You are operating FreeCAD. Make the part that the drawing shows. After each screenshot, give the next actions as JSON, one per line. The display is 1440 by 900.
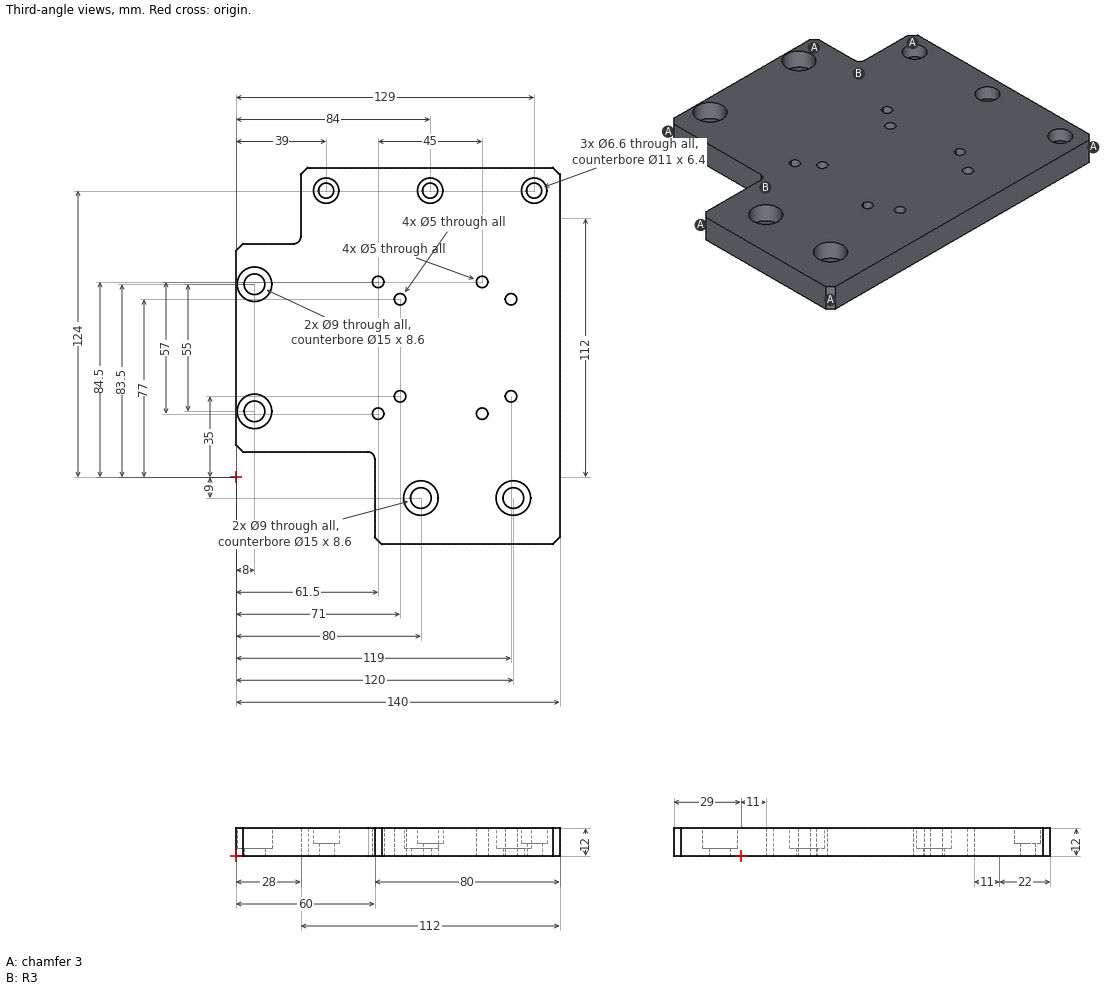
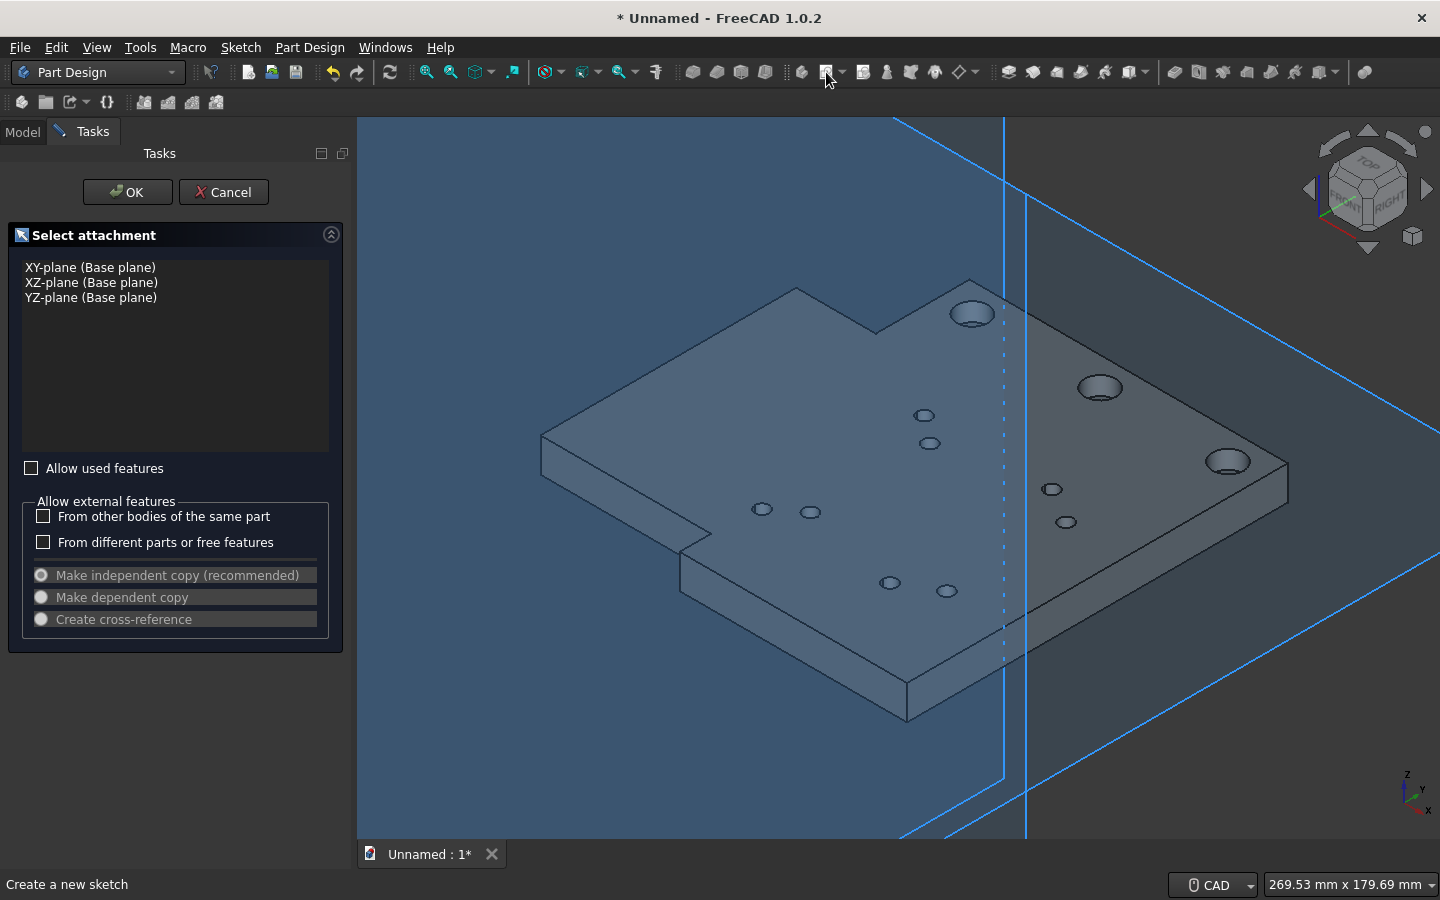
{"action": "left_click", "coordinate": [82, 282]}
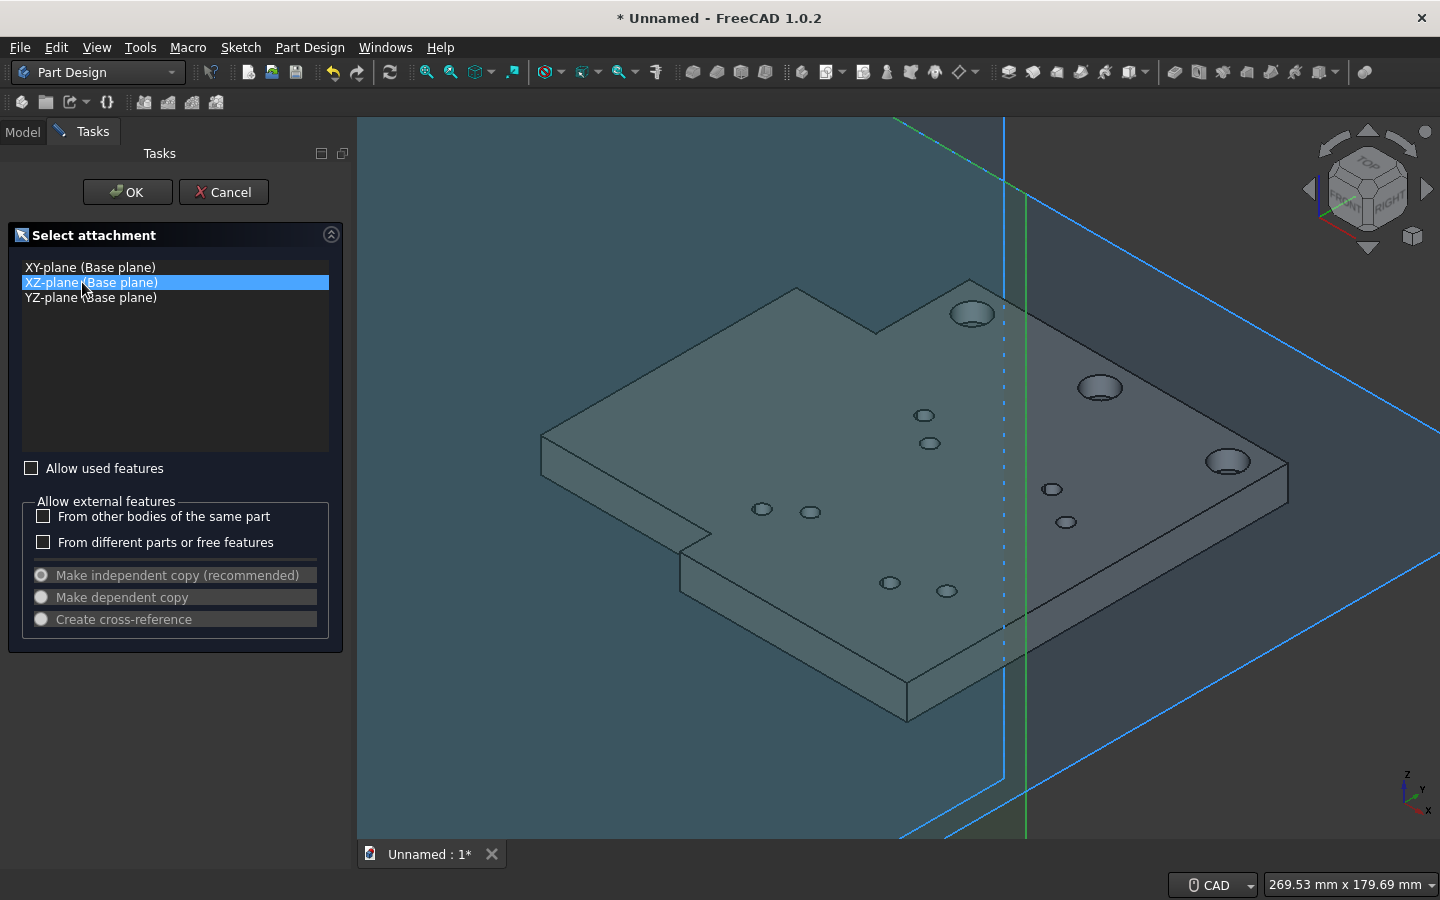
{"action": "left_click", "coordinate": [128, 192]}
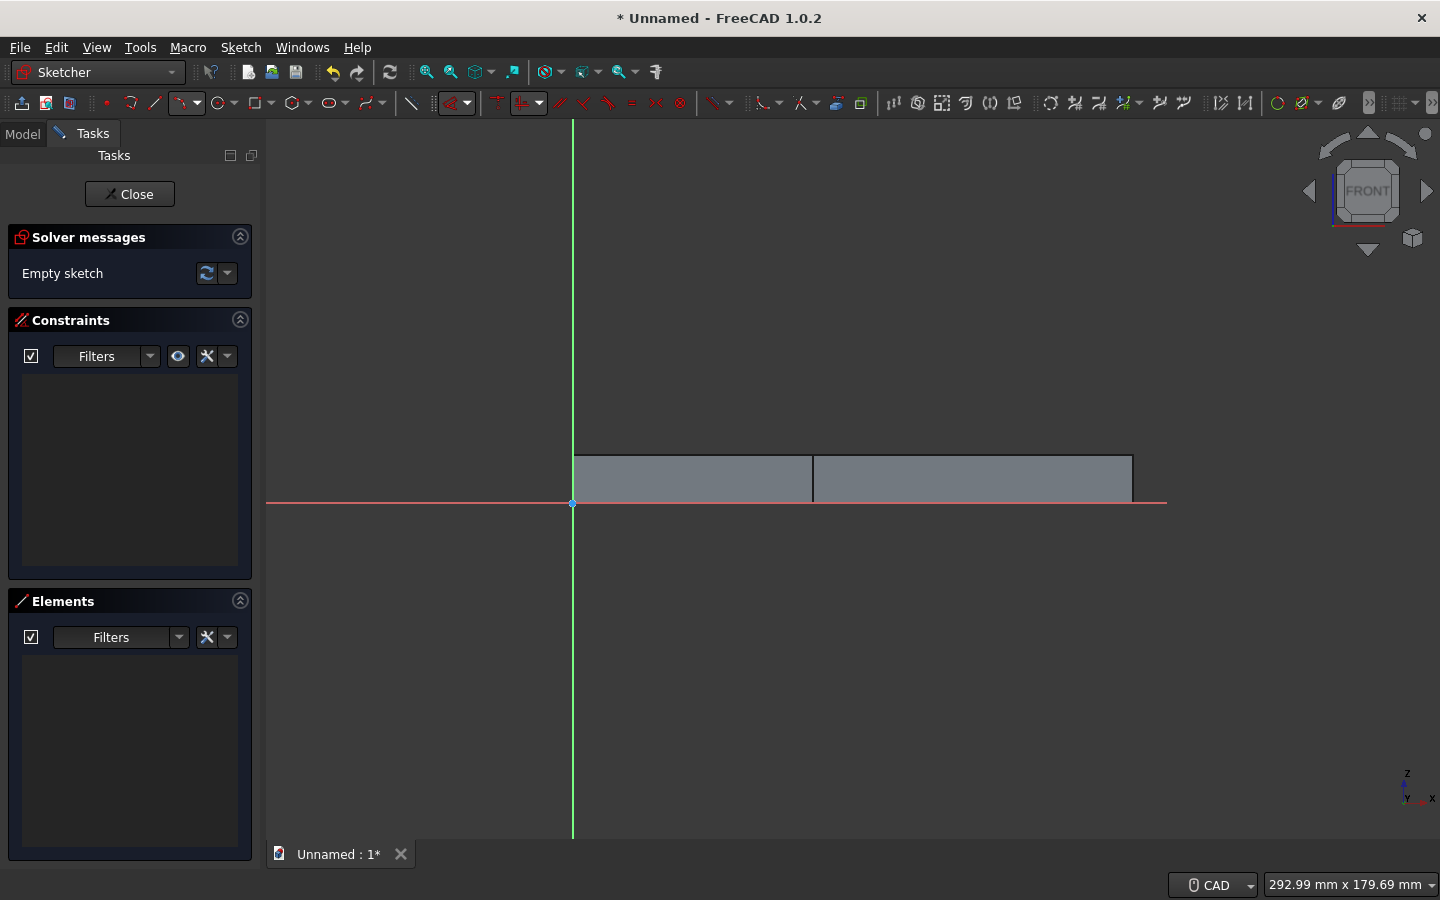
{"action": "left_click", "coordinate": [256, 104]}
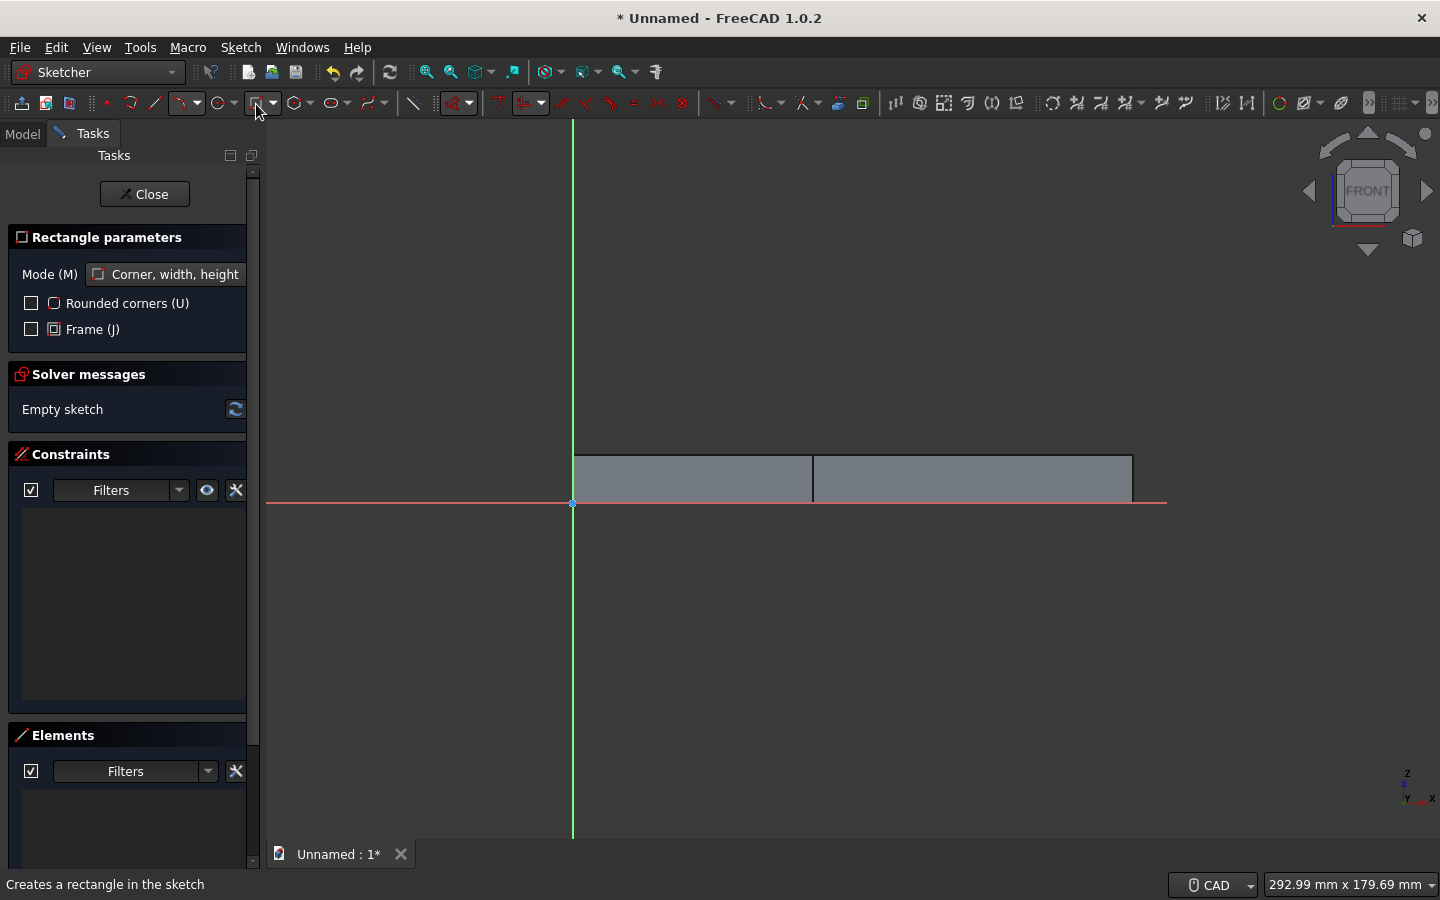
{"action": "left_click", "coordinate": [813, 455]}
{"action": "left_click", "coordinate": [1133, 503]}
{"action": "key", "text": "Escape"}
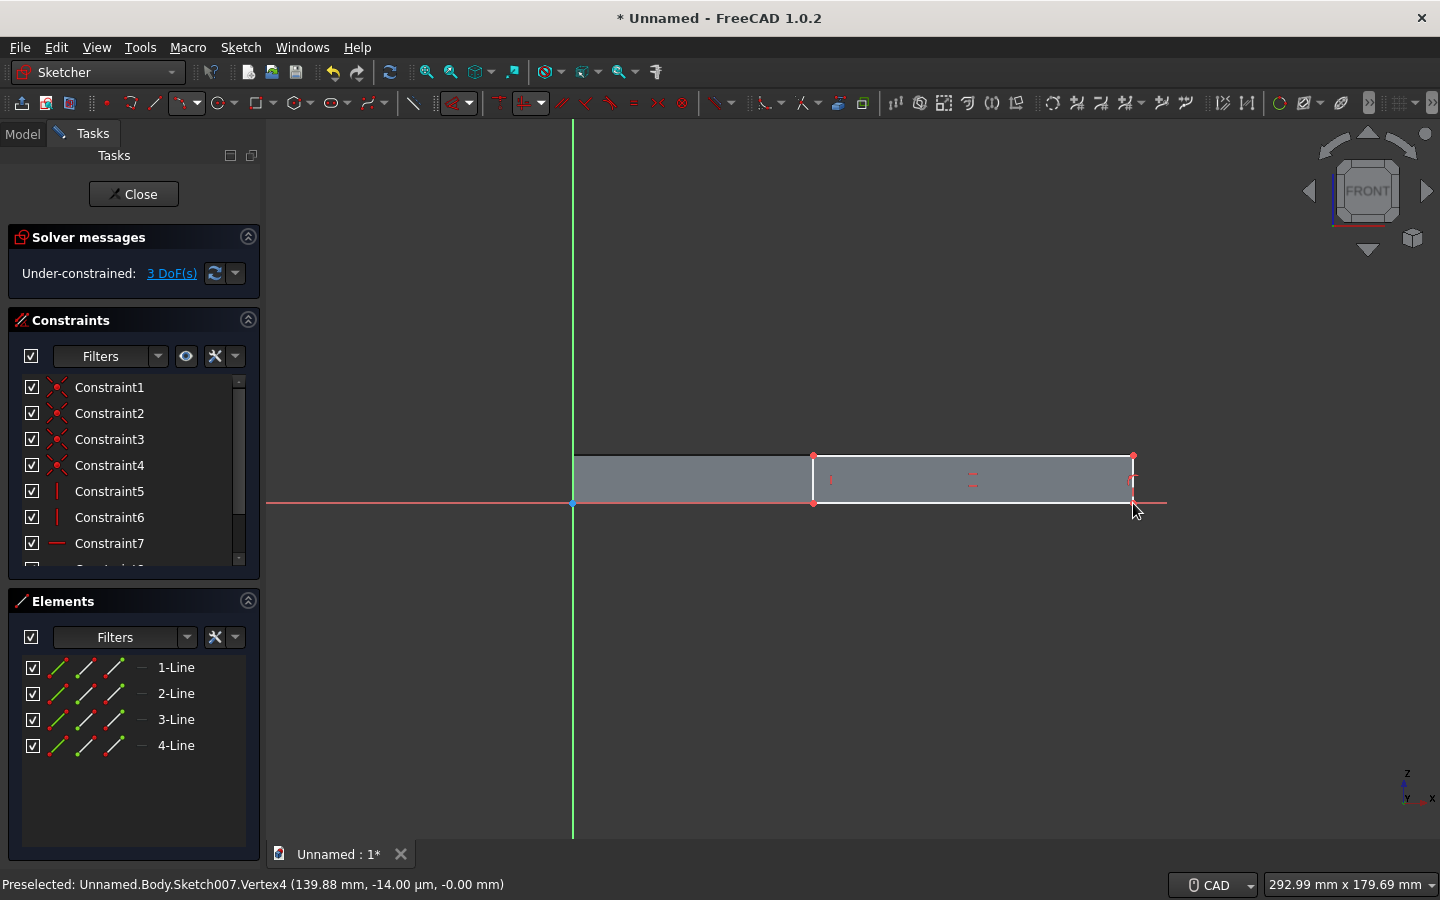
{"action": "left_click", "coordinate": [813, 470]}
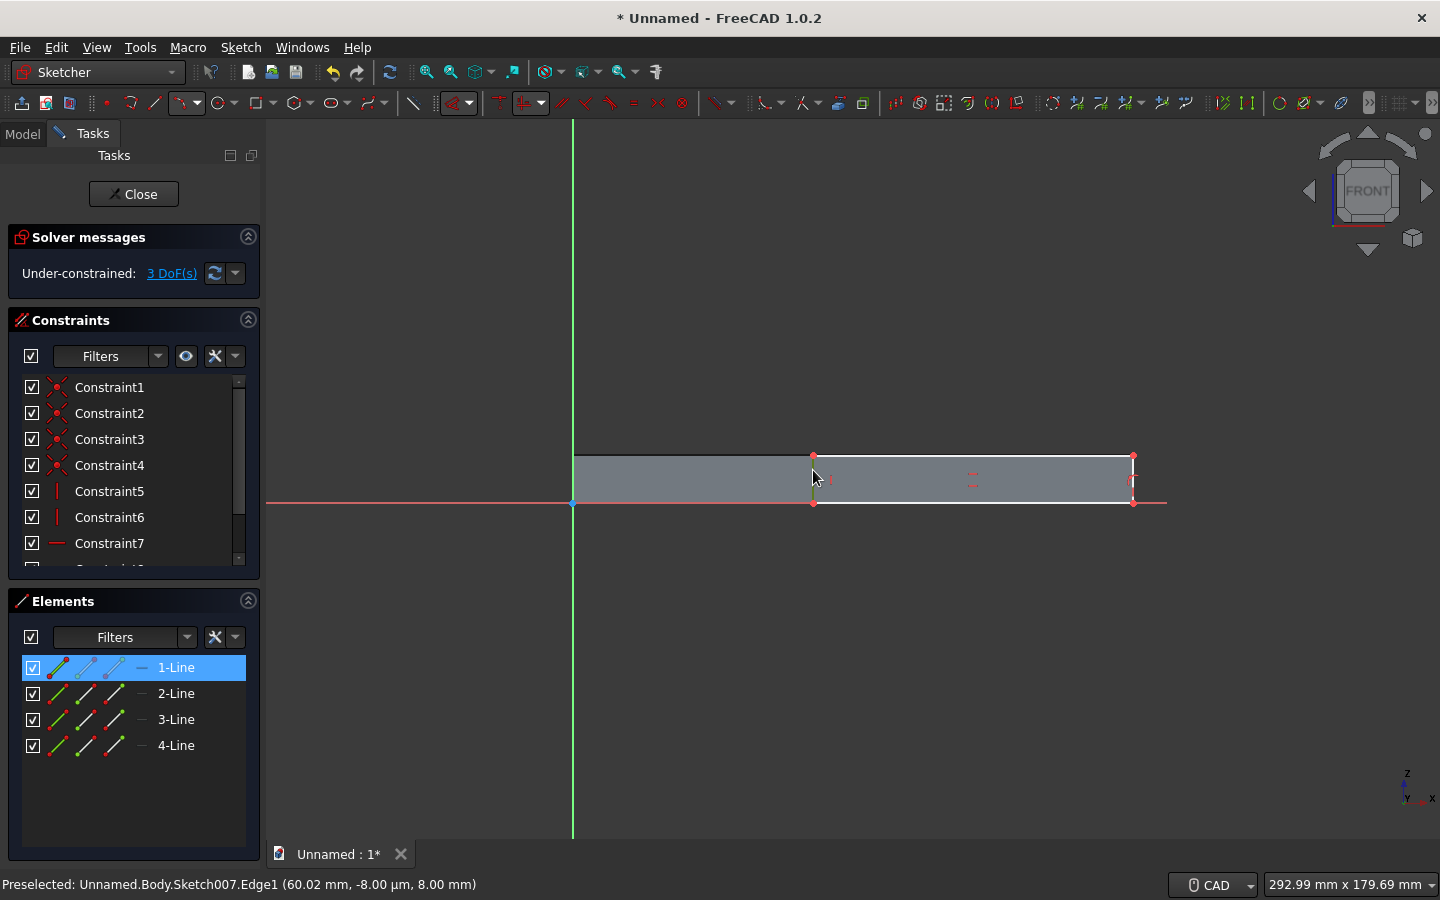
{"action": "key", "text": "i"}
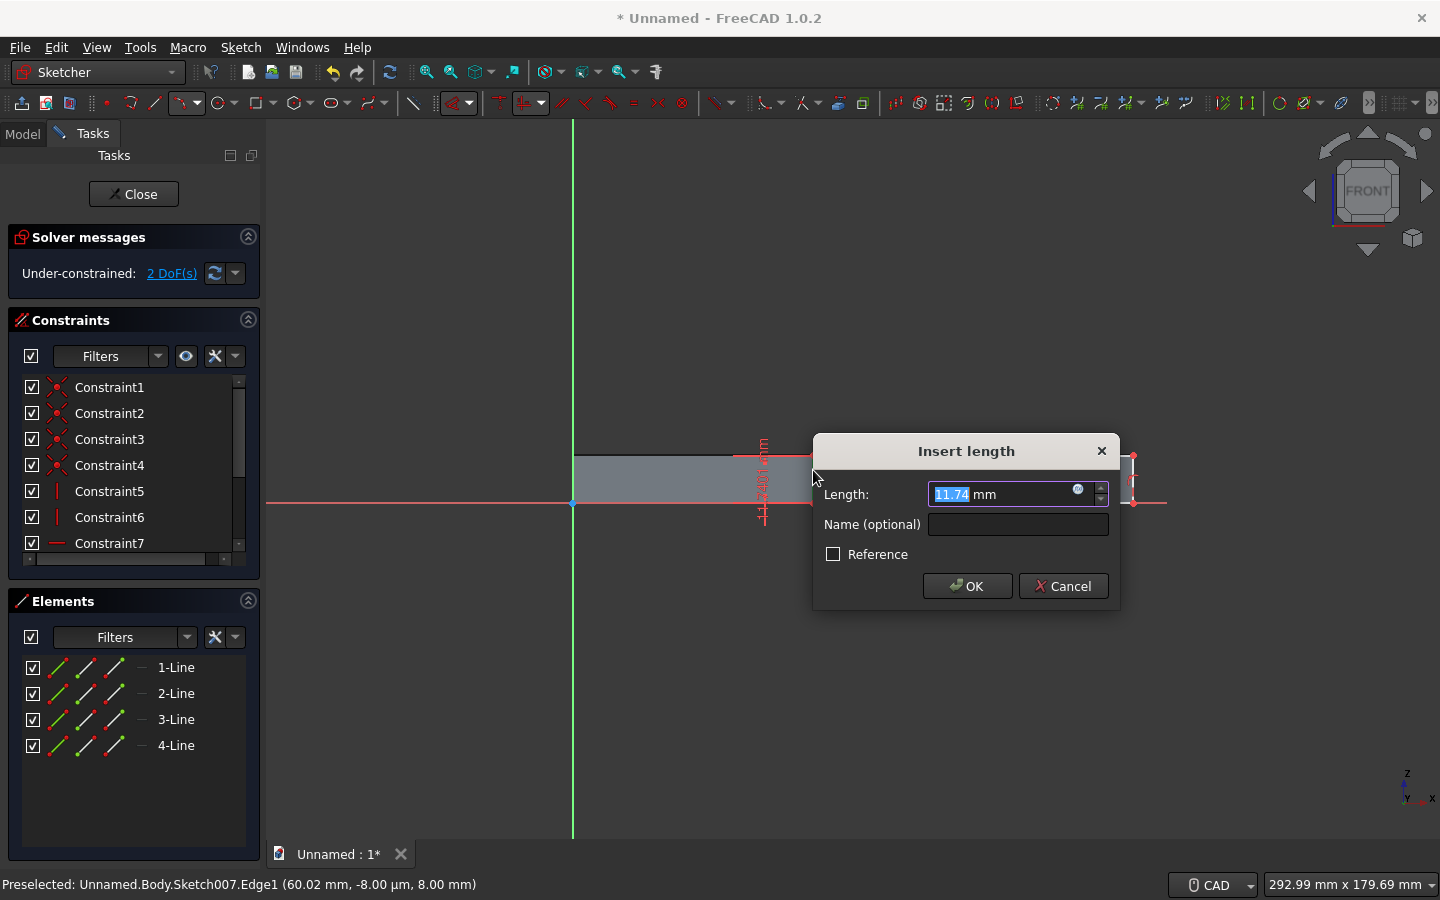
{"action": "type", "text": "12"}
{"action": "key", "text": "Return"}